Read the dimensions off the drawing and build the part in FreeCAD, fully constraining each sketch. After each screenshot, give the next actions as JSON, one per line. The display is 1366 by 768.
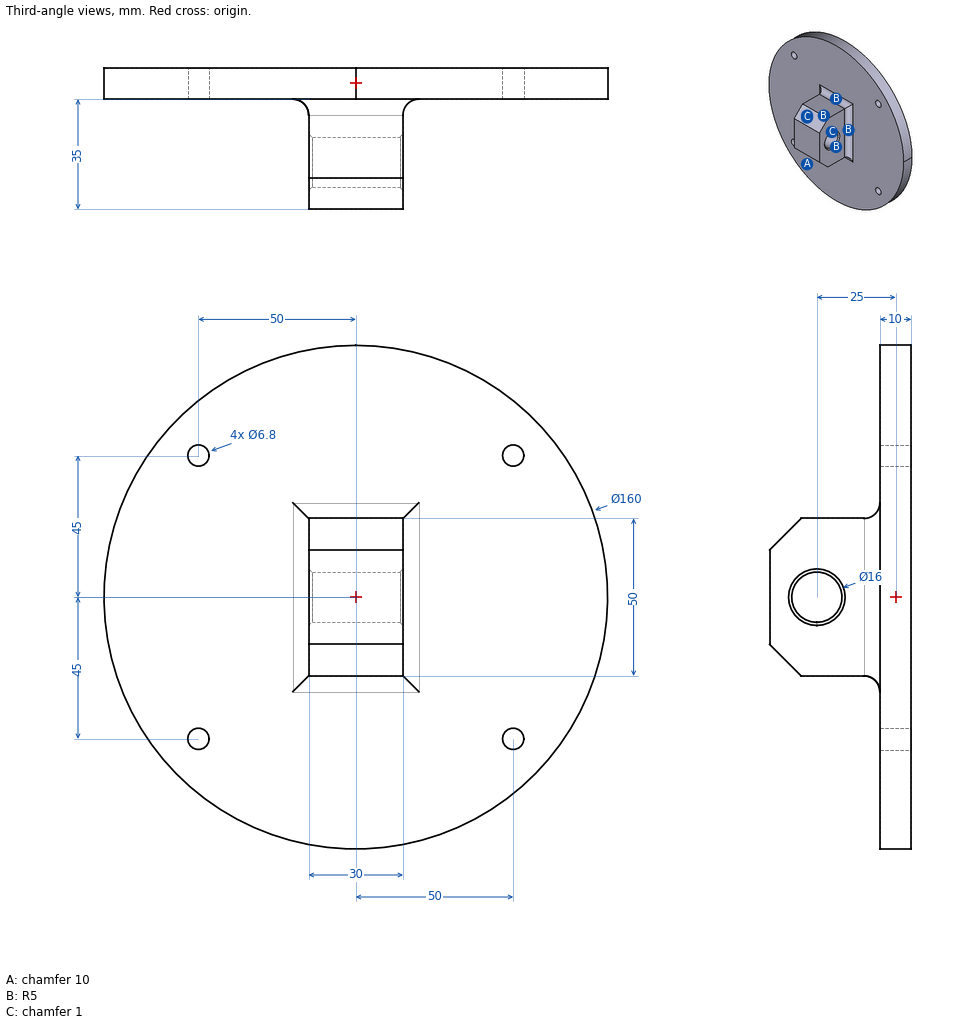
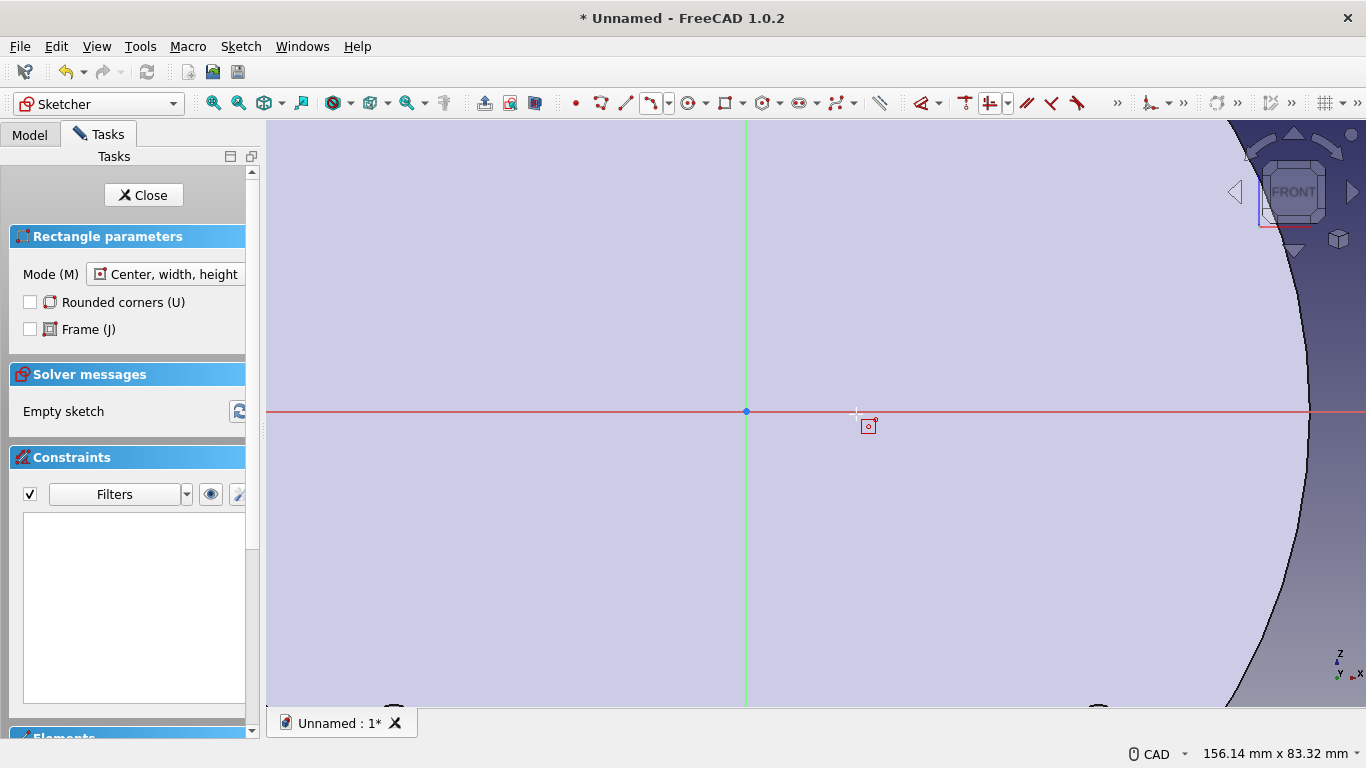
{"action": "left_click", "coordinate": [746, 412]}
{"action": "left_click", "coordinate": [852, 236]}
{"action": "key", "text": "Escape"}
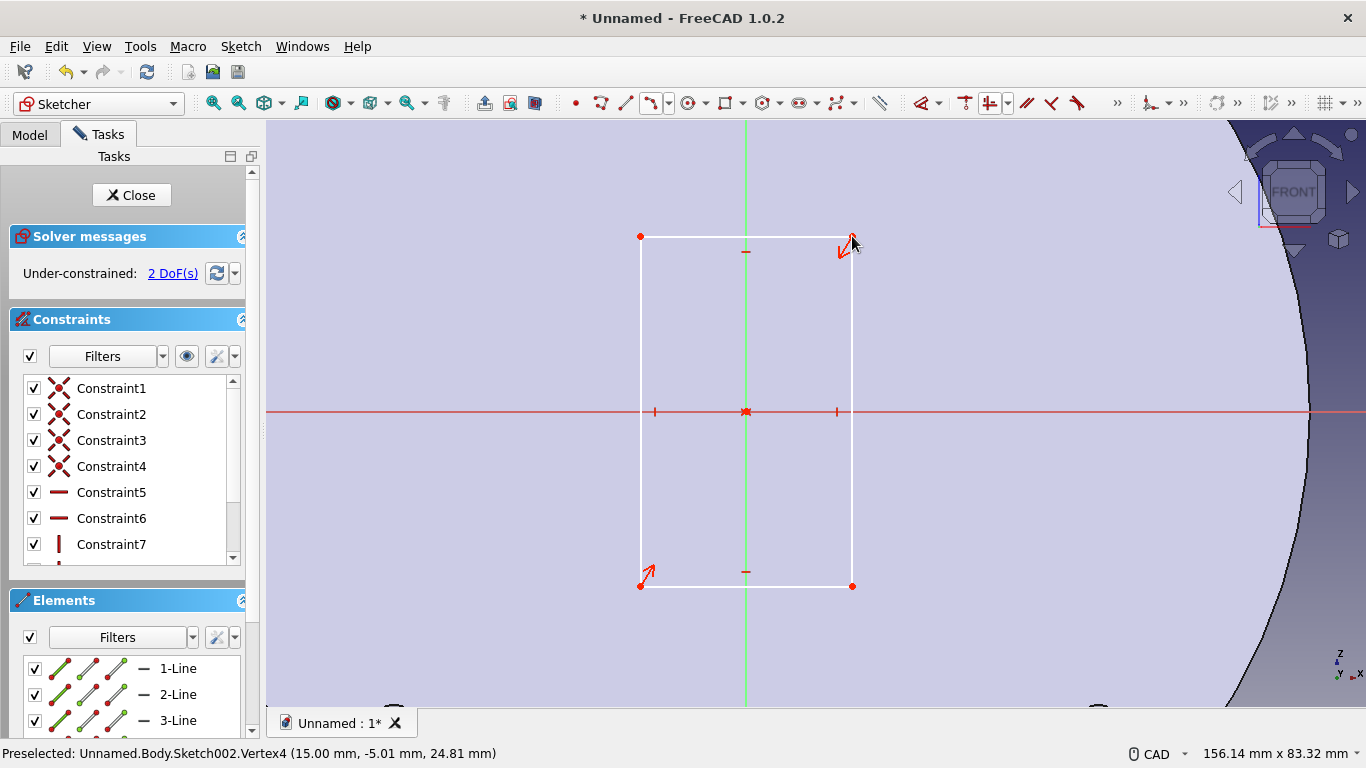
{"action": "key", "text": "d"}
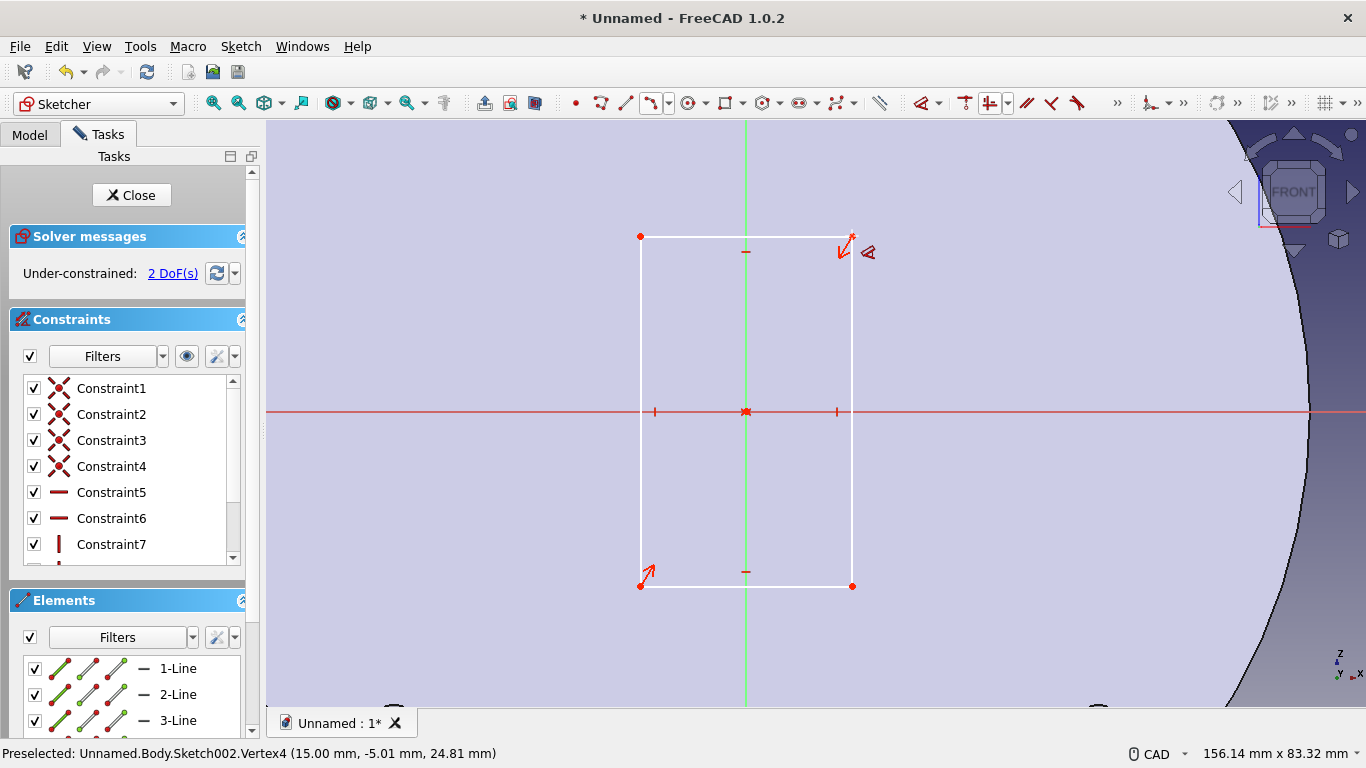
{"action": "left_click", "coordinate": [704, 587]}
{"action": "left_click", "coordinate": [698, 621]}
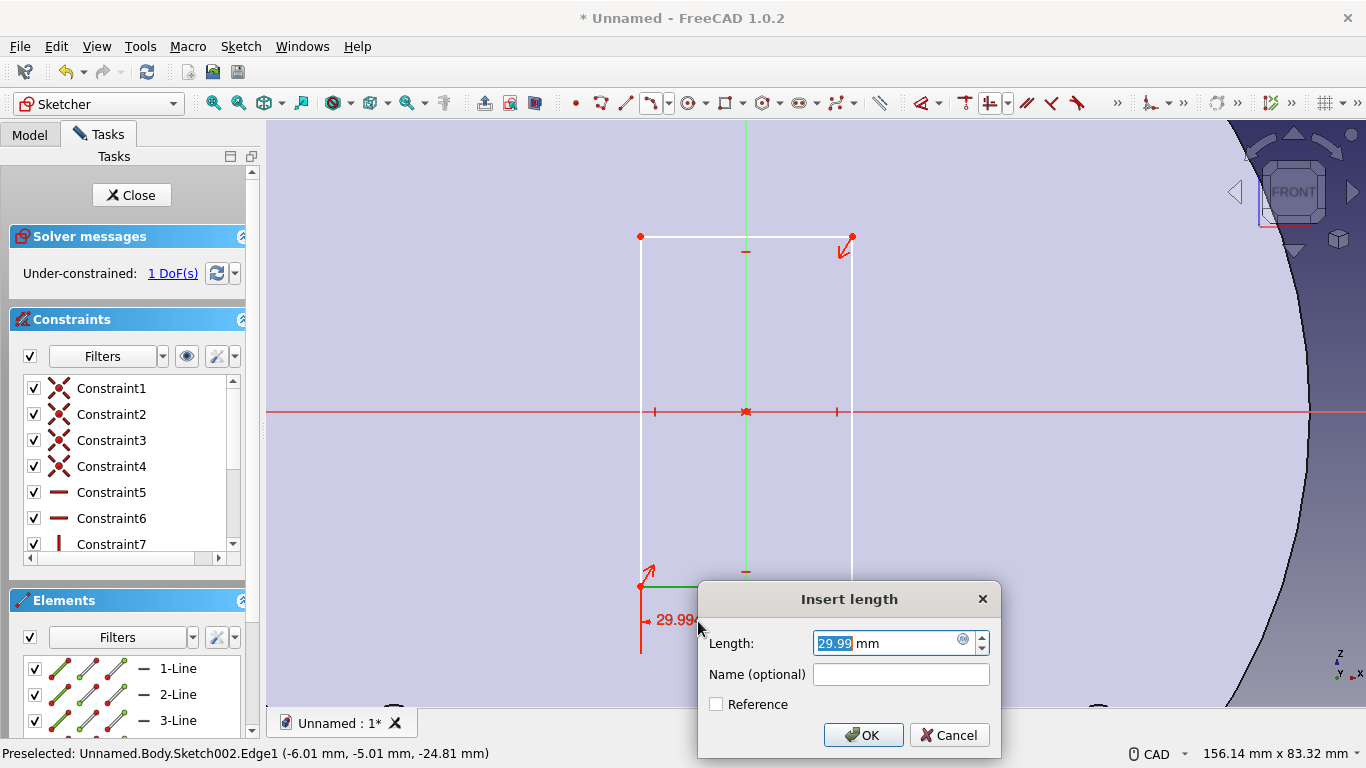
{"action": "type", "text": "30"}
{"action": "key", "text": "Return"}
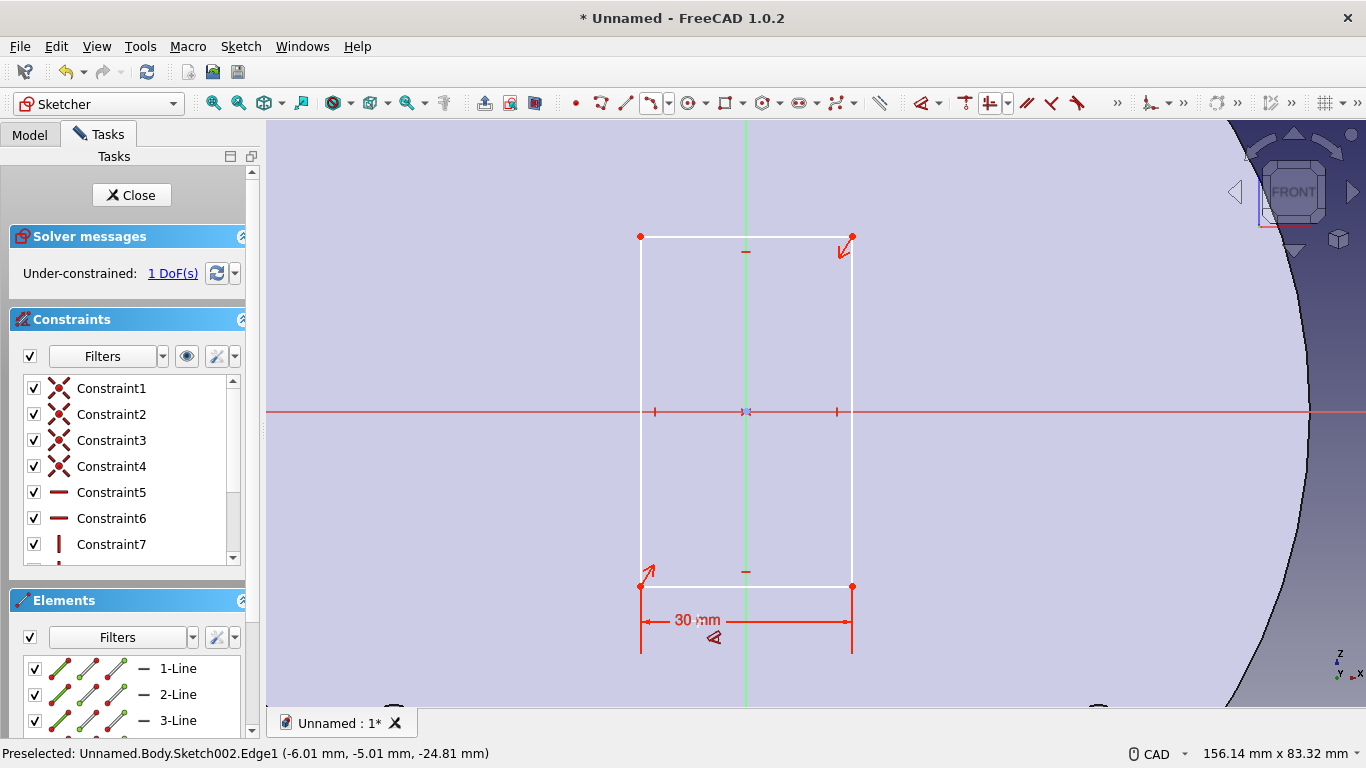
{"action": "left_click", "coordinate": [852, 482]}
{"action": "left_click", "coordinate": [886, 331]}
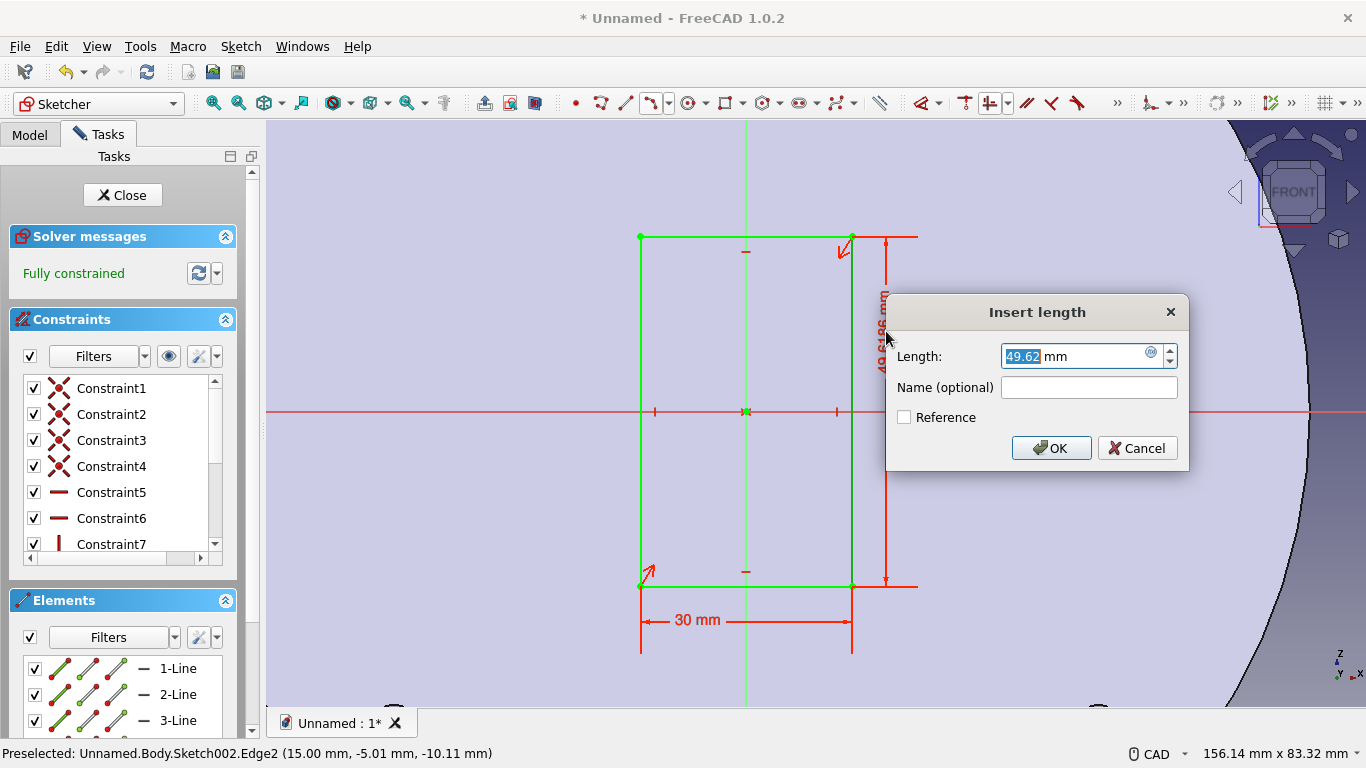
{"action": "type", "text": "50"}
{"action": "key", "text": "Return"}
{"action": "key", "text": "Escape"}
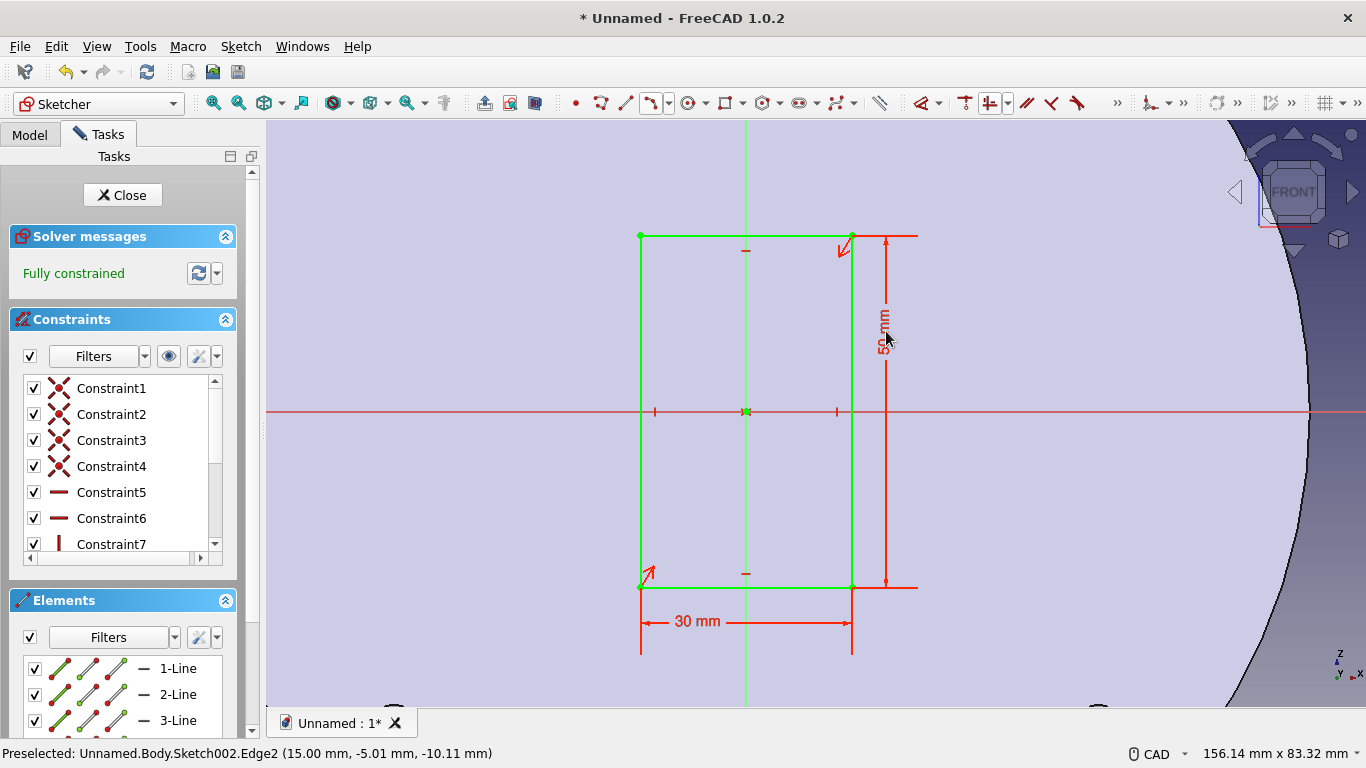
{"action": "left_click", "coordinate": [123, 195]}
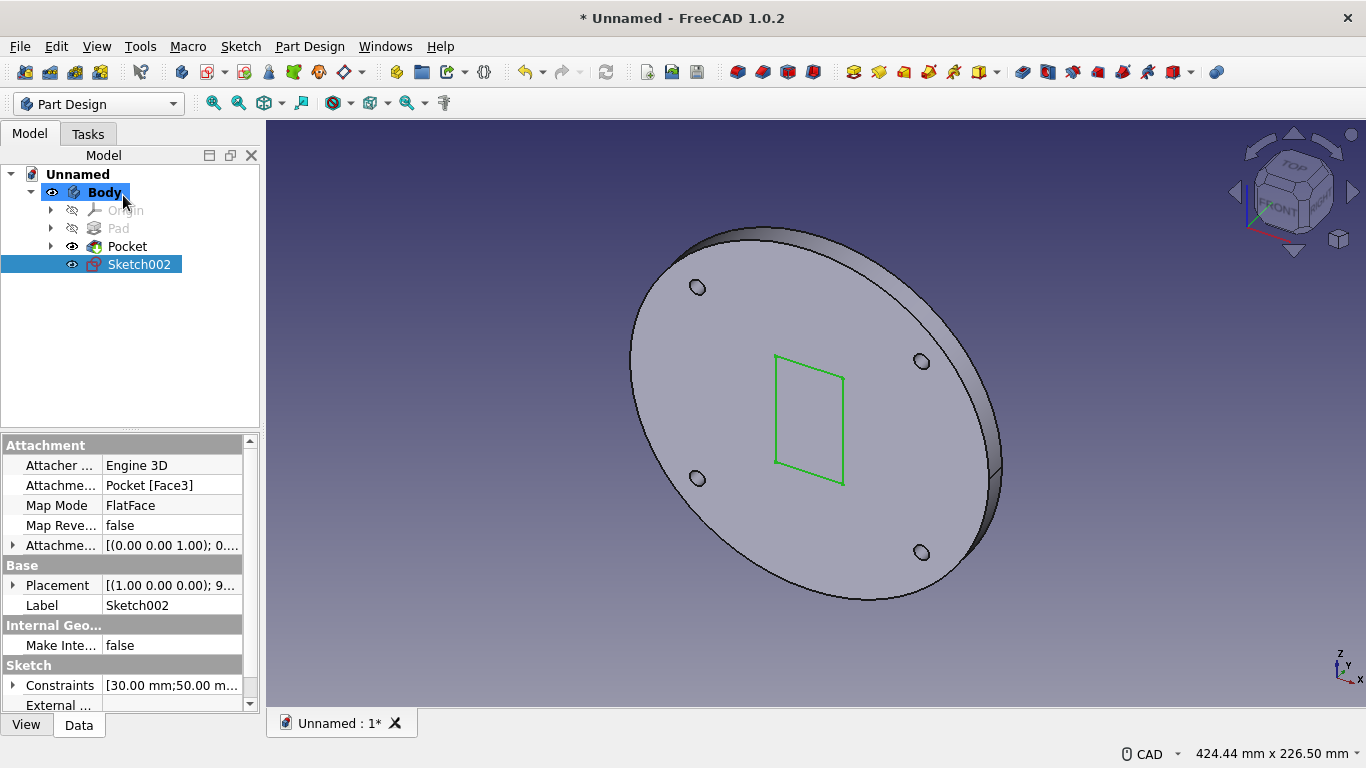
{"action": "left_click", "coordinate": [854, 72]}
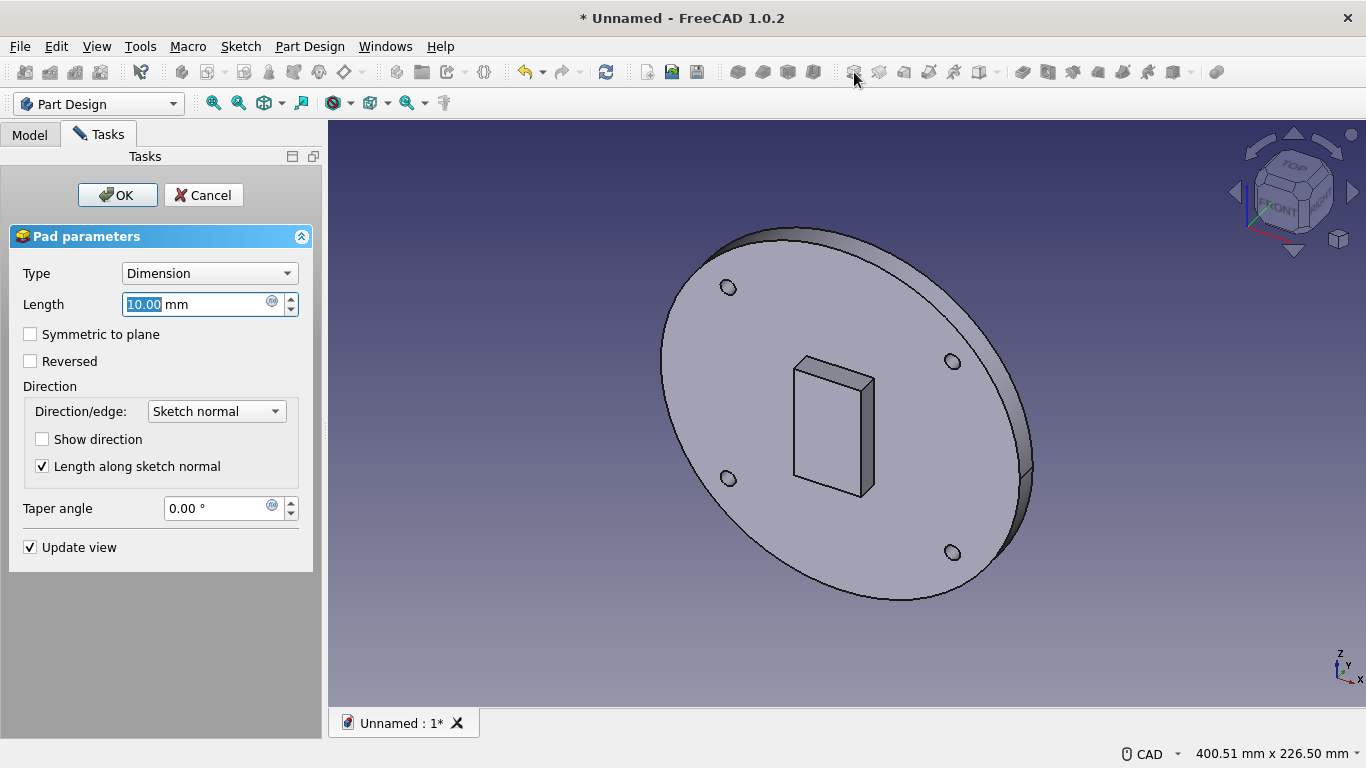
{"action": "type", "text": "35"}
{"action": "key", "text": "Tab"}